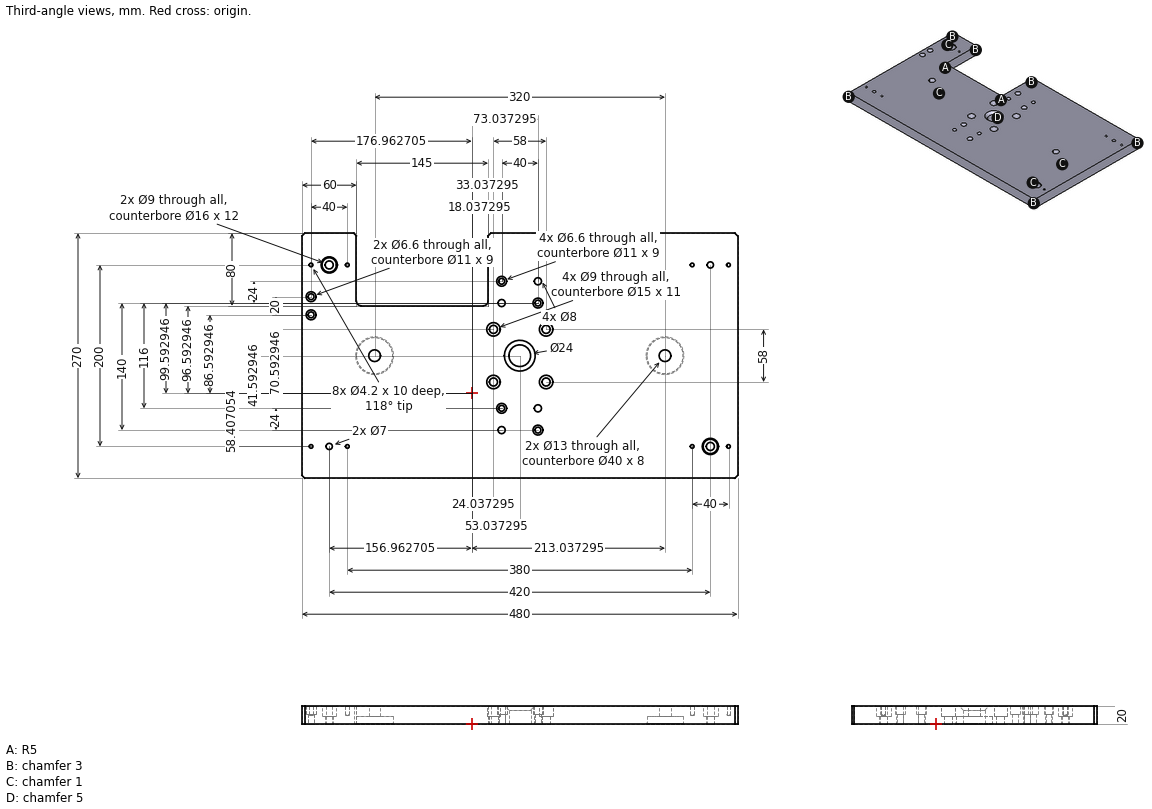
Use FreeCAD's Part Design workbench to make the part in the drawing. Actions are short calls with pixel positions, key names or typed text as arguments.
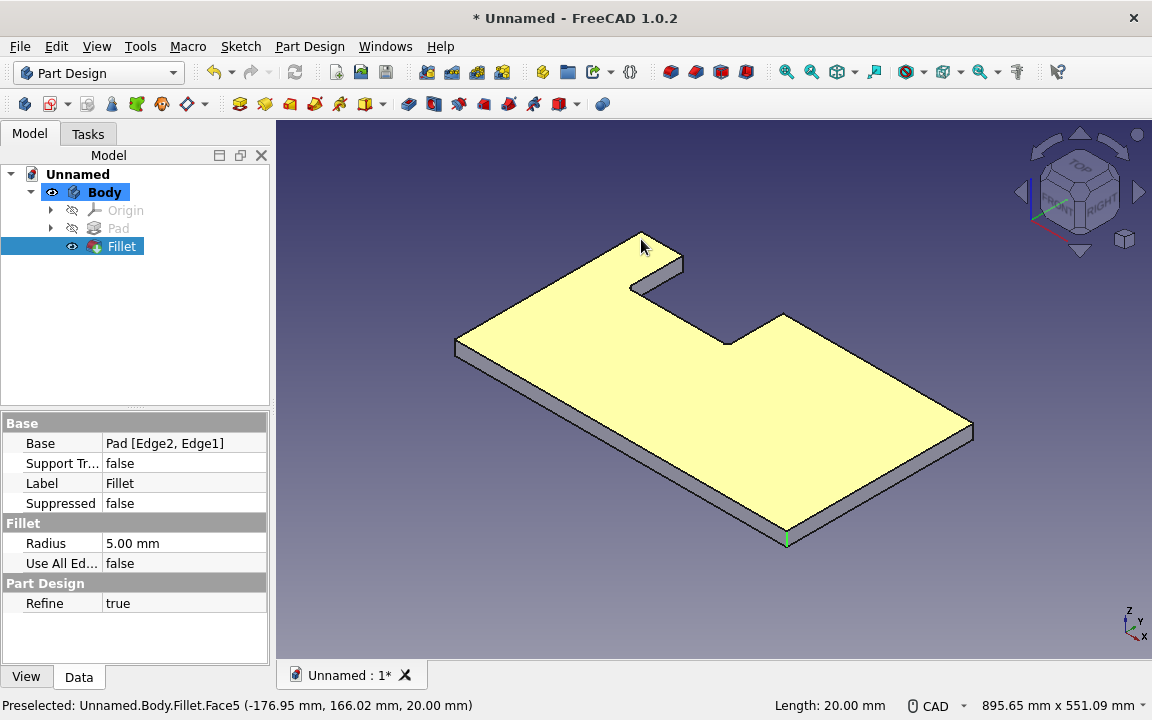
key(1)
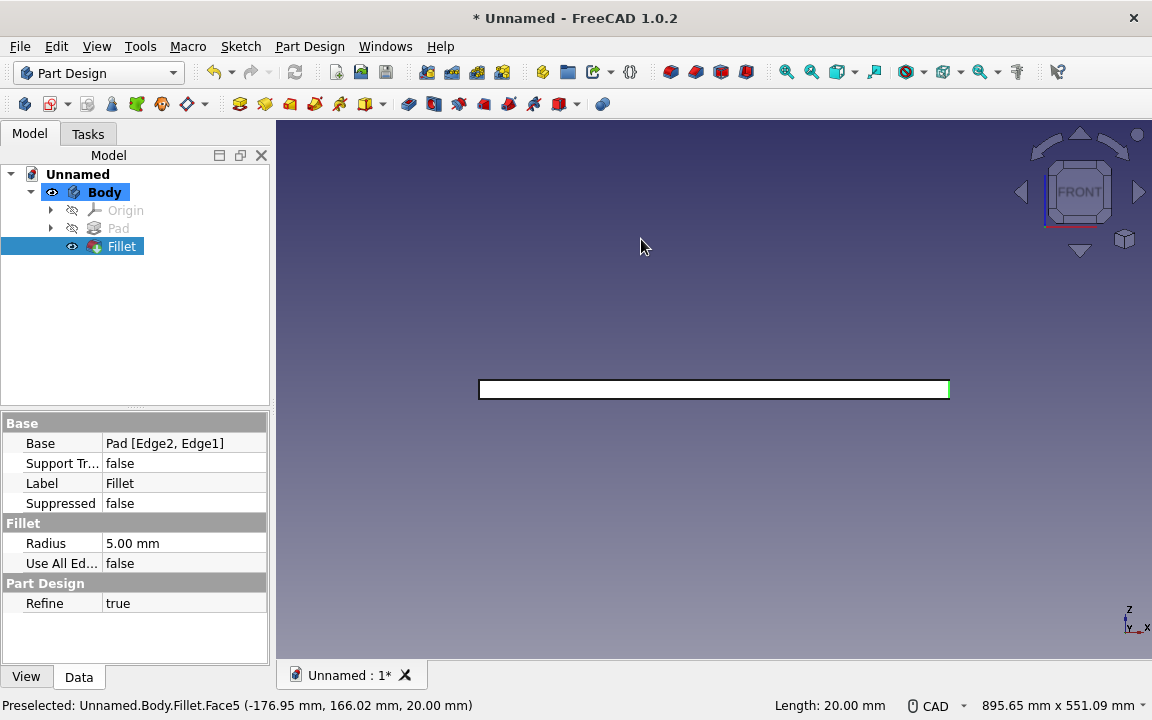
click(479, 388, ctrl)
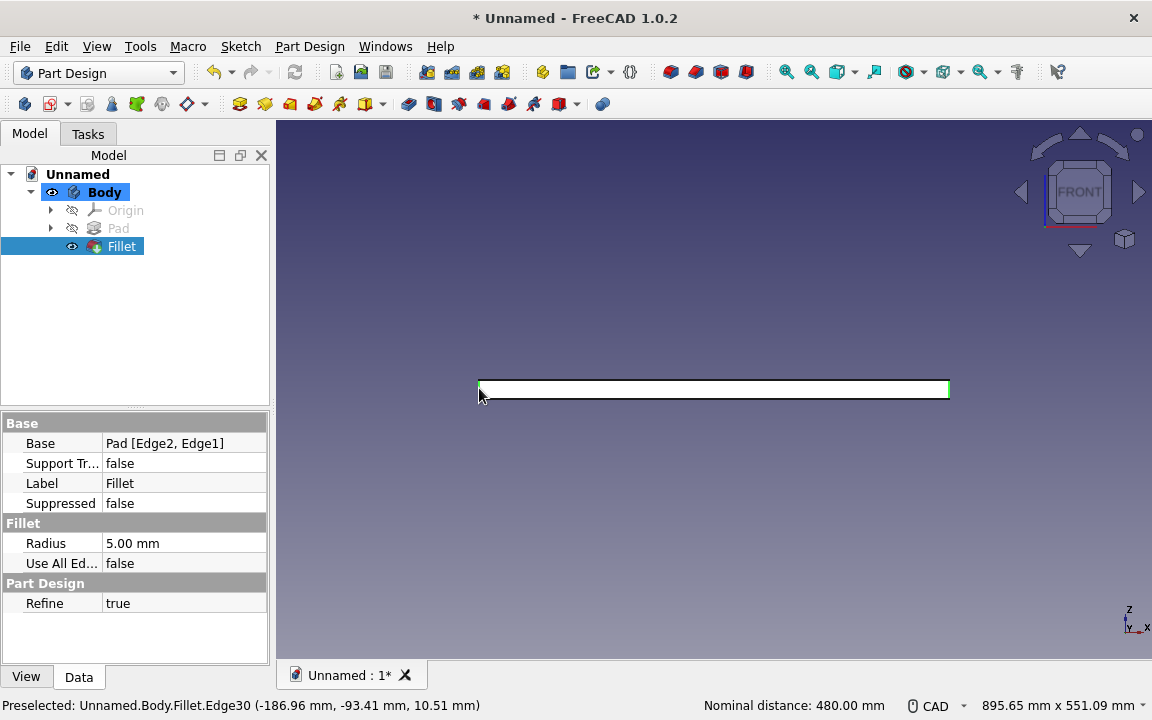
scroll(479, 388, up, 4)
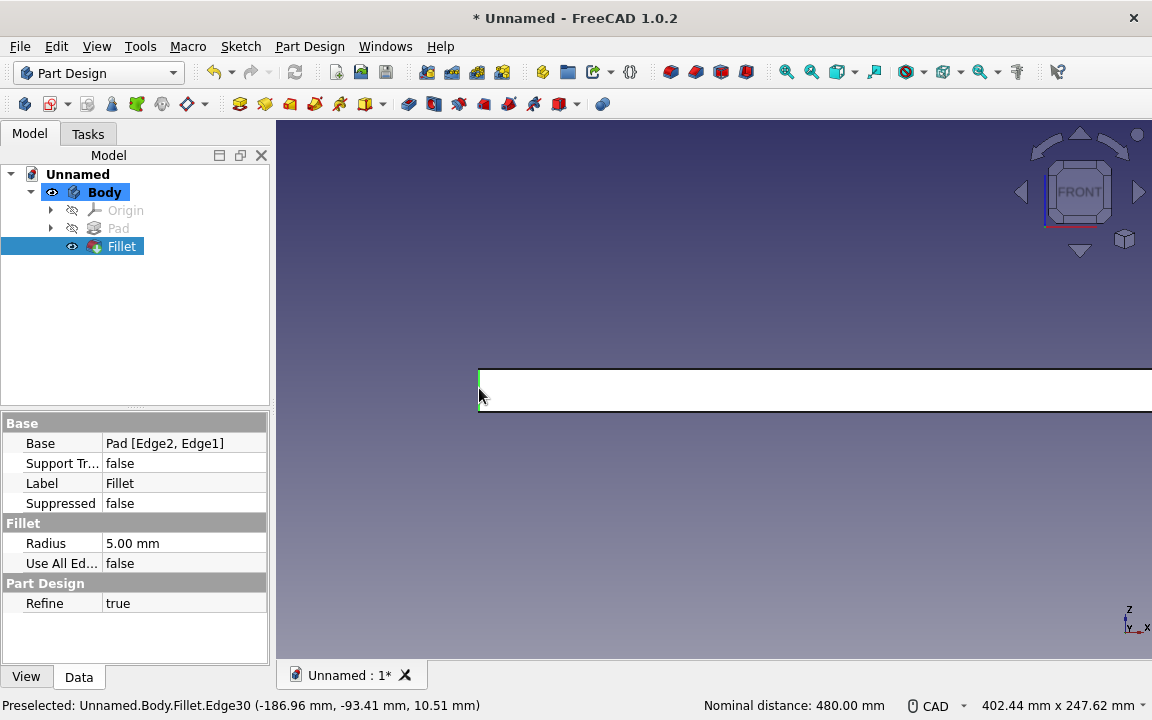
key(v)
key(f)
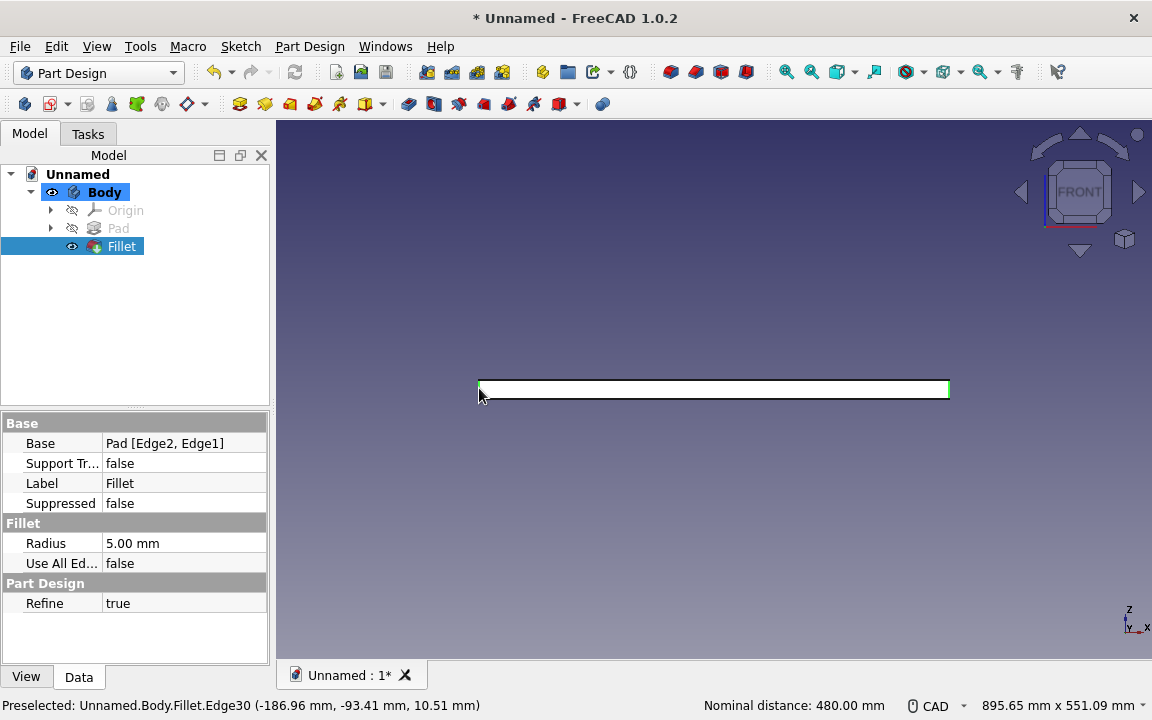
key(3)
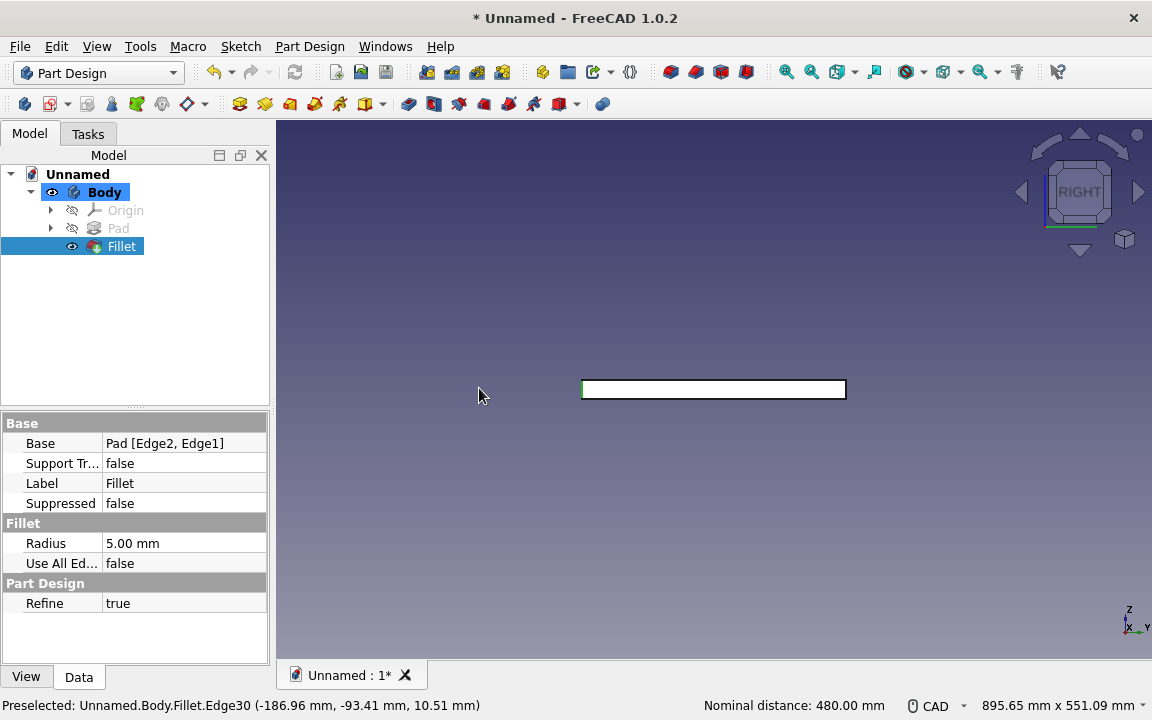
key(v)
key(f)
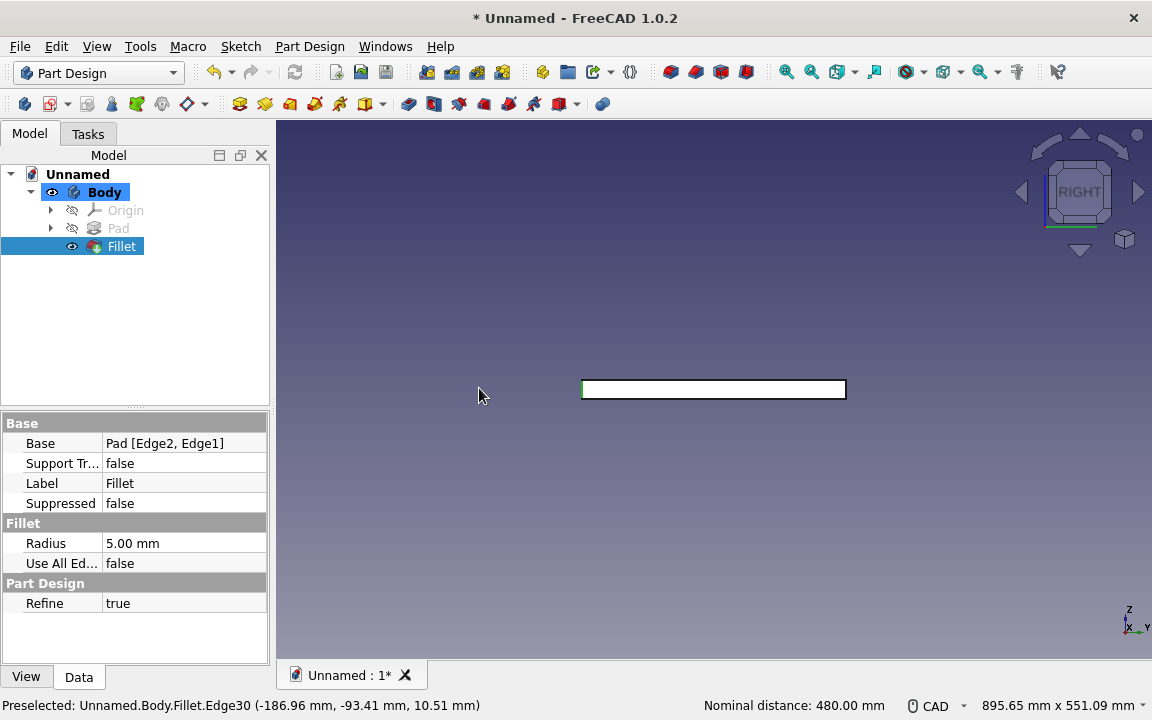
click(846, 388, ctrl)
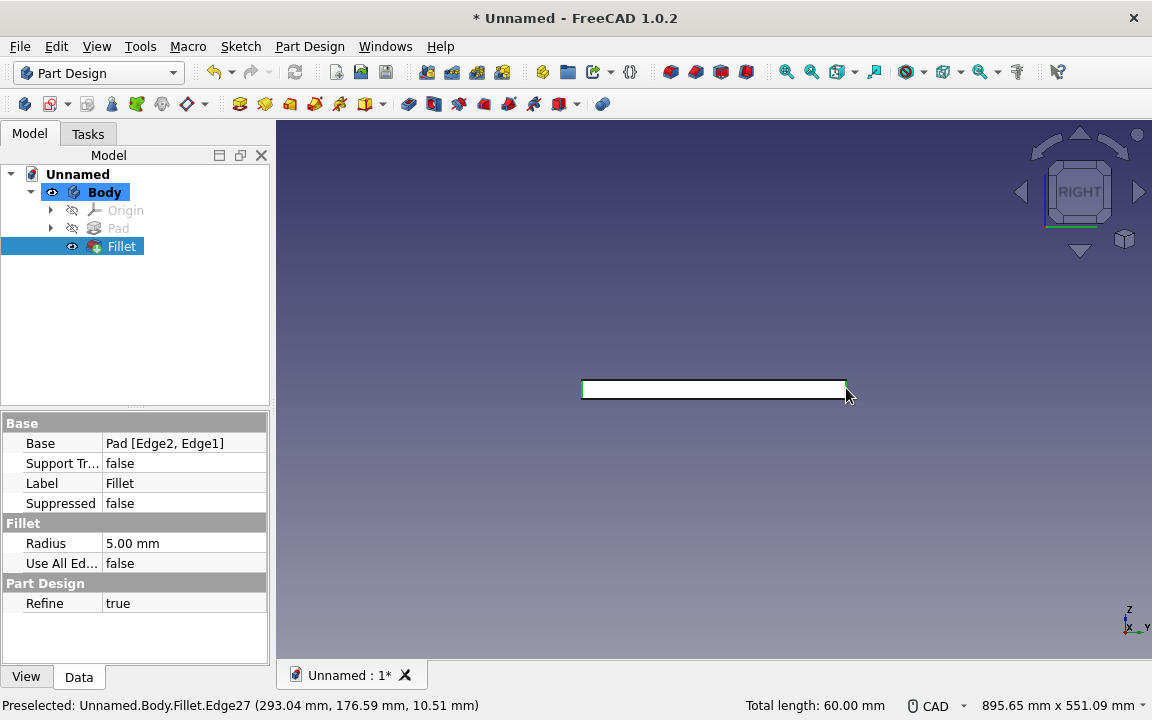
scroll(846, 388, up, 4)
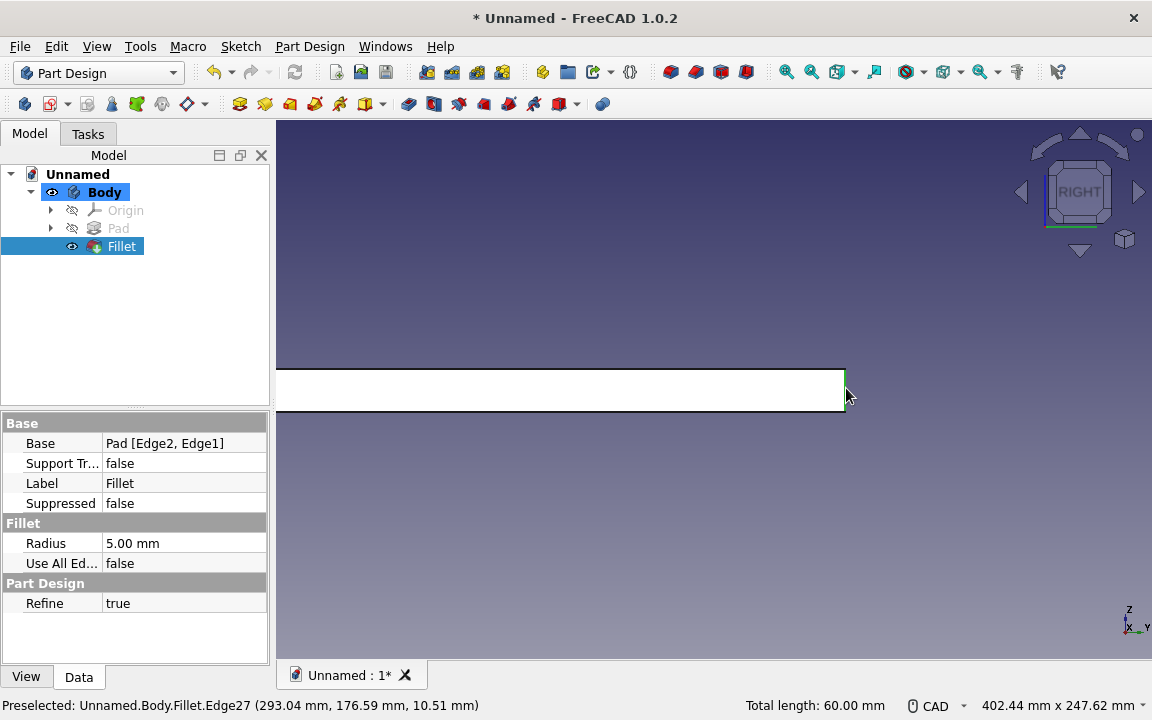
click(787, 72)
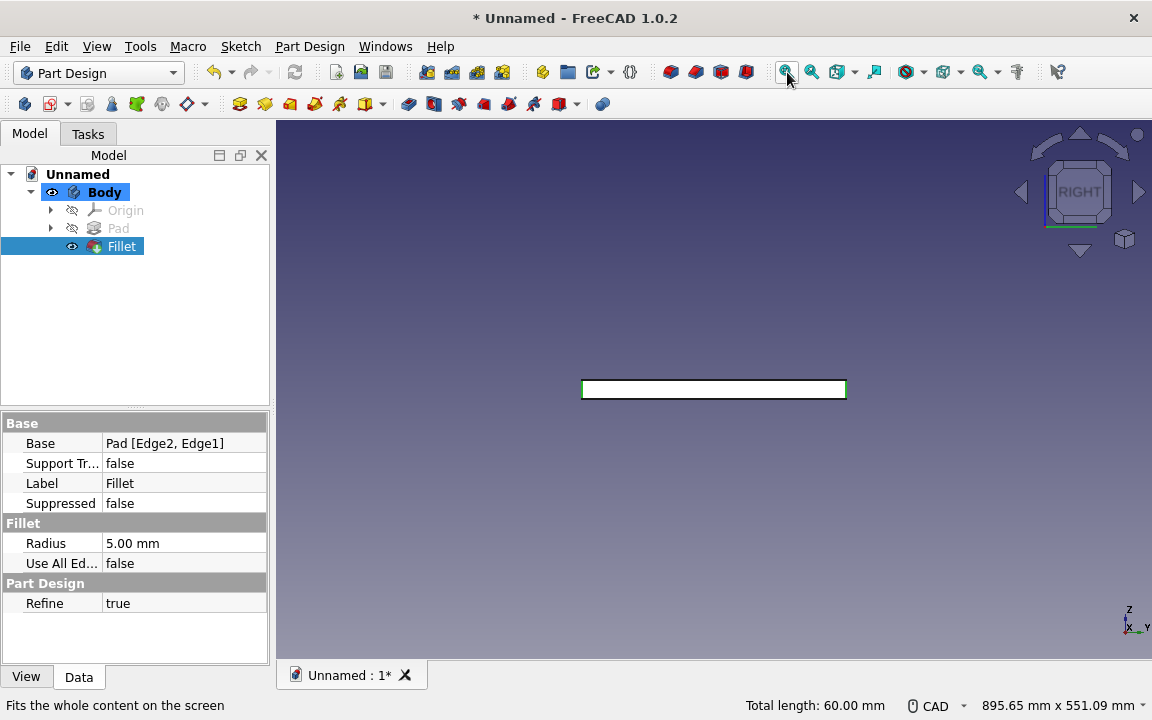
key(5)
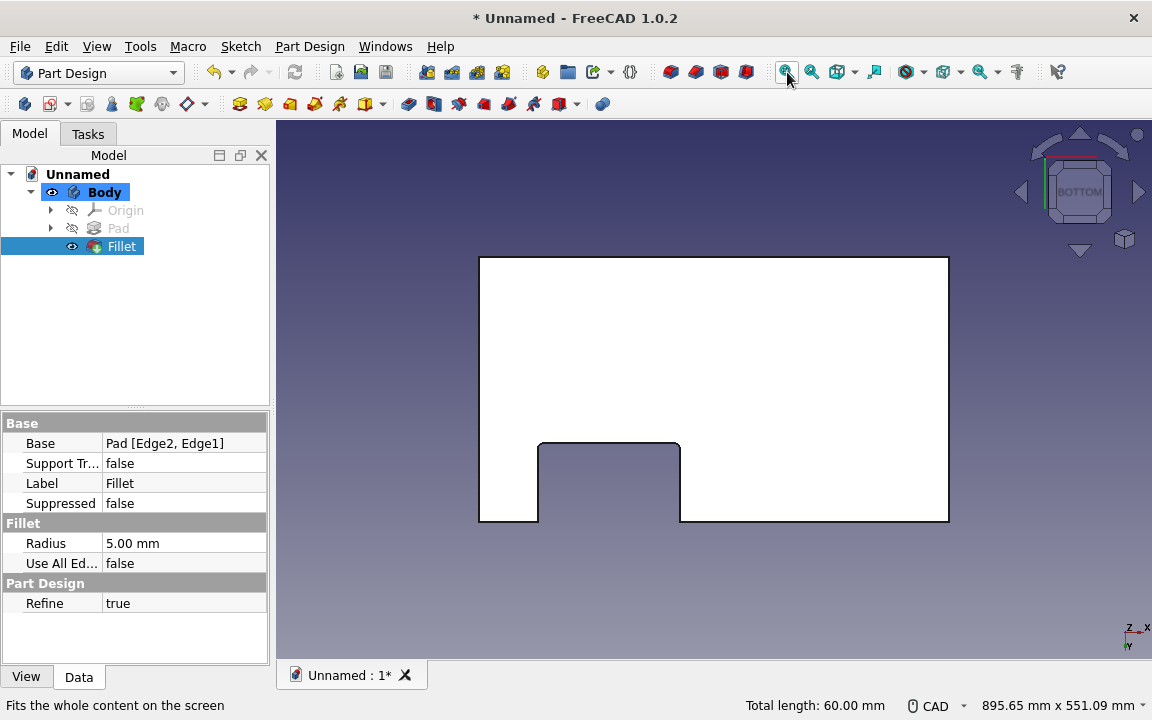
scroll(479, 521, up, 4)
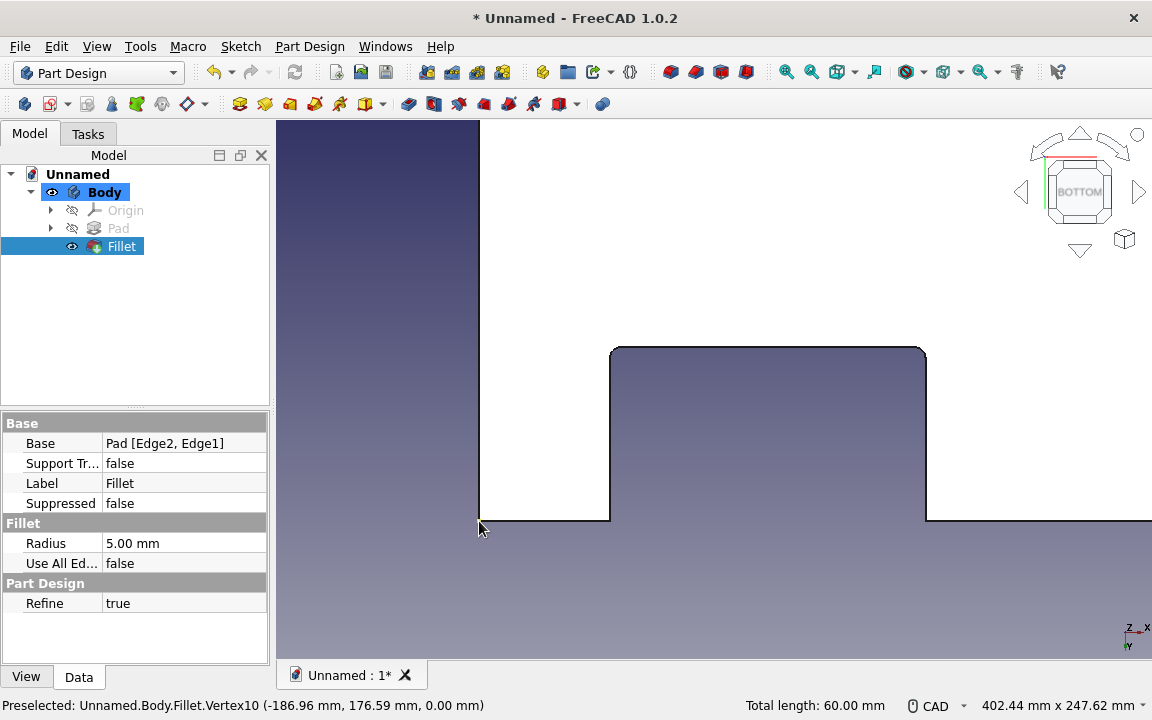
key(v)
key(f)